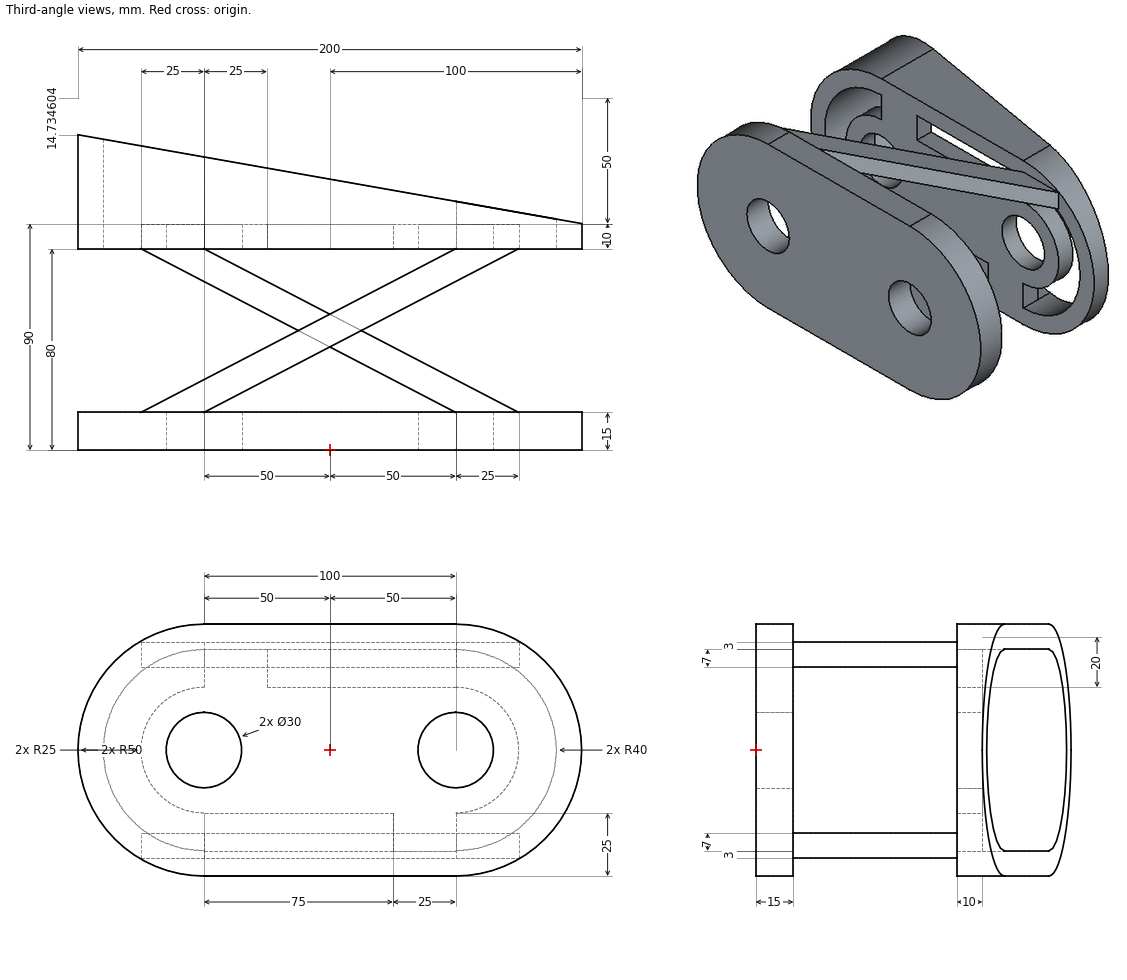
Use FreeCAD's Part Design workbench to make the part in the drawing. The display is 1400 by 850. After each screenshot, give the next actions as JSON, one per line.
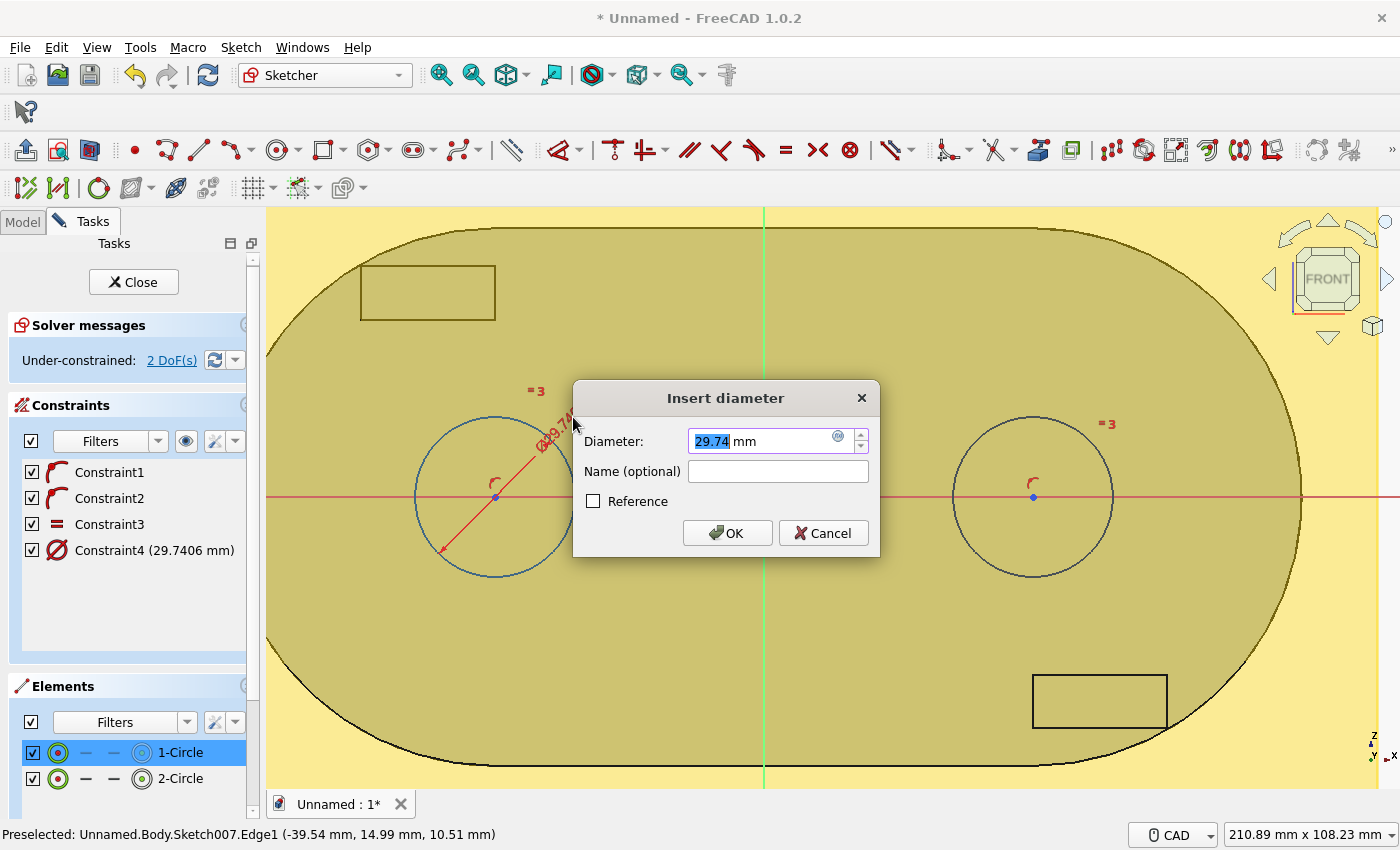
{"action": "type", "text": "30"}
{"action": "key", "text": "Return"}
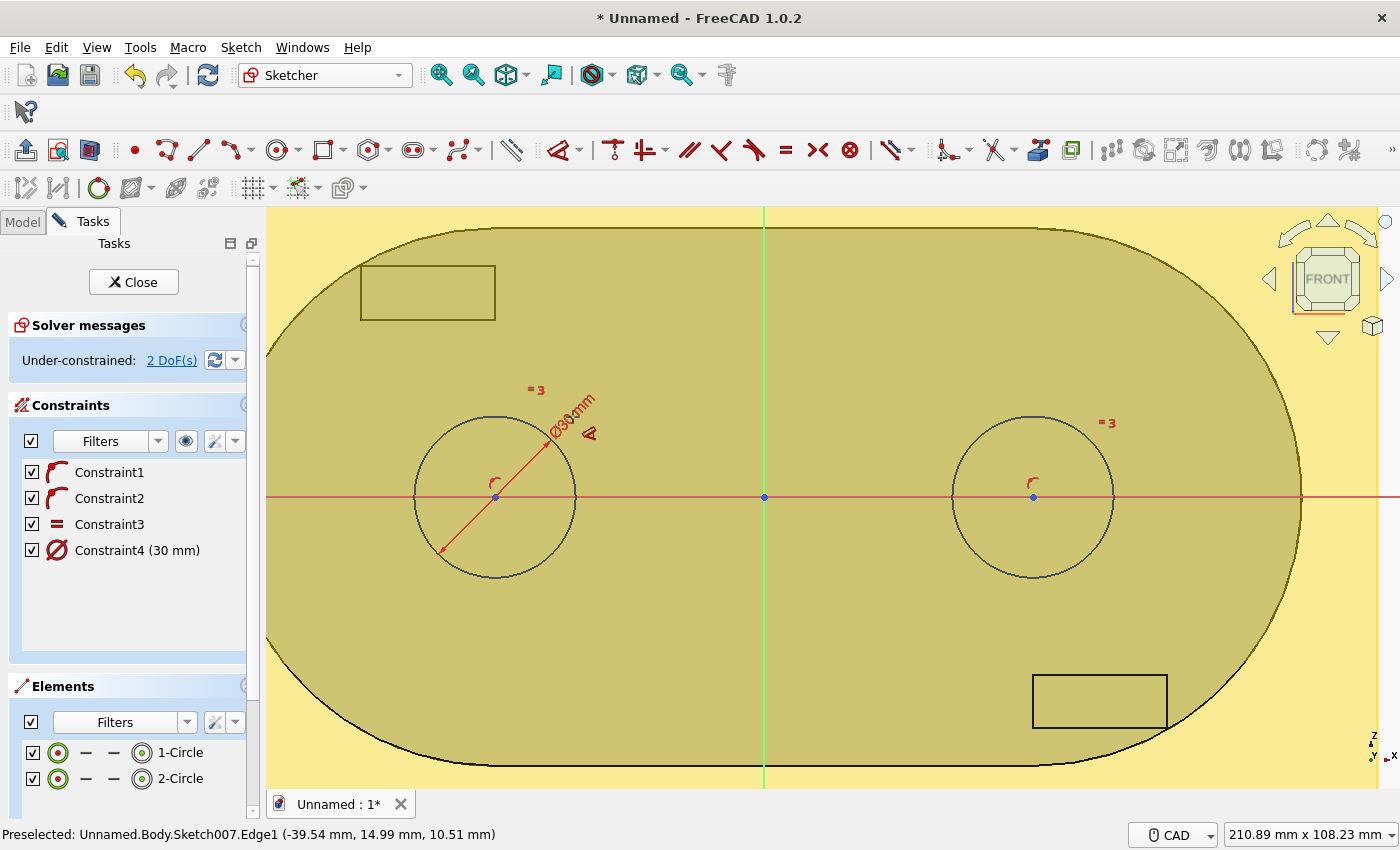
{"action": "left_click", "coordinate": [495, 497]}
{"action": "left_click", "coordinate": [630, 531]}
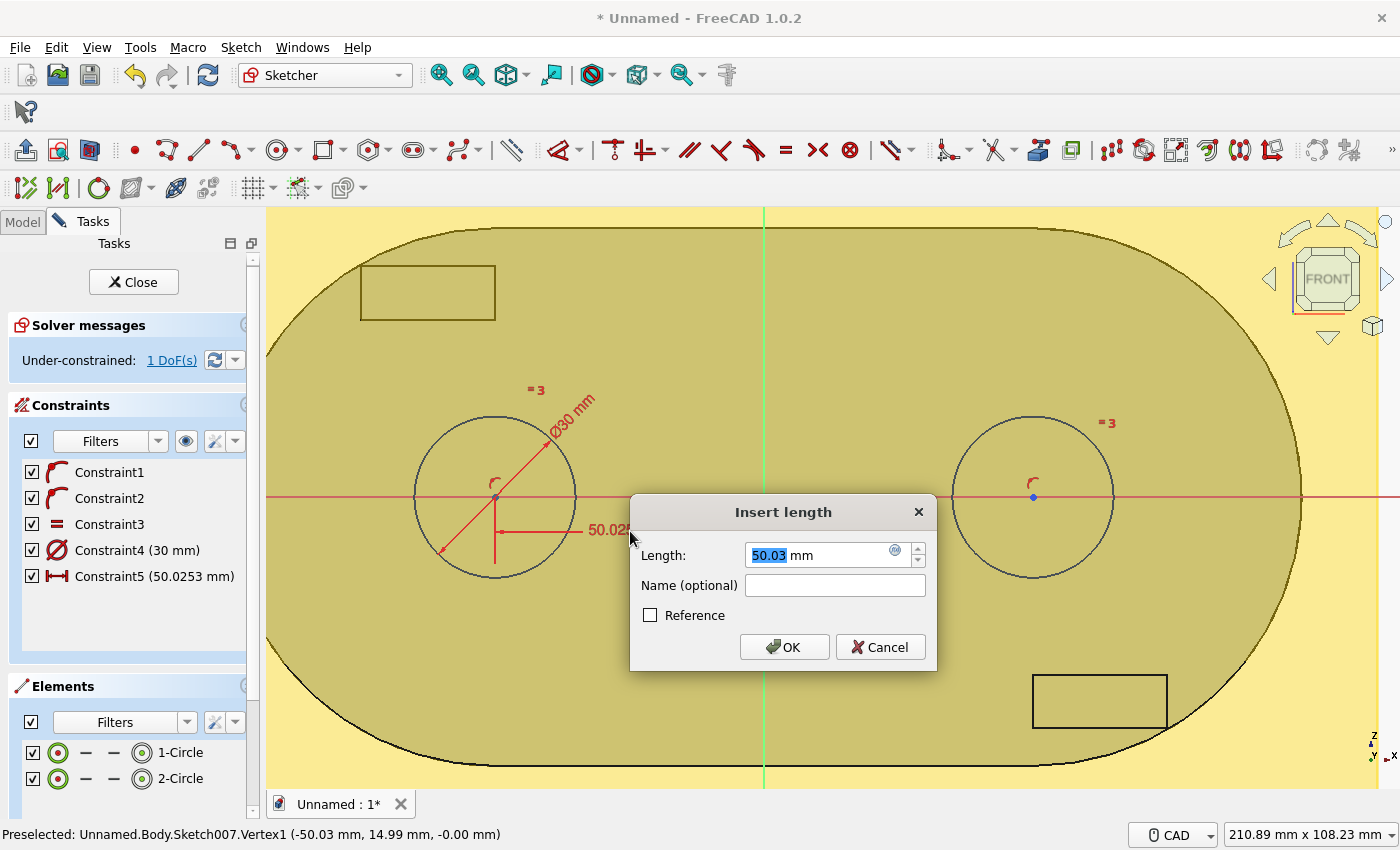
{"action": "type", "text": "50"}
{"action": "key", "text": "Return"}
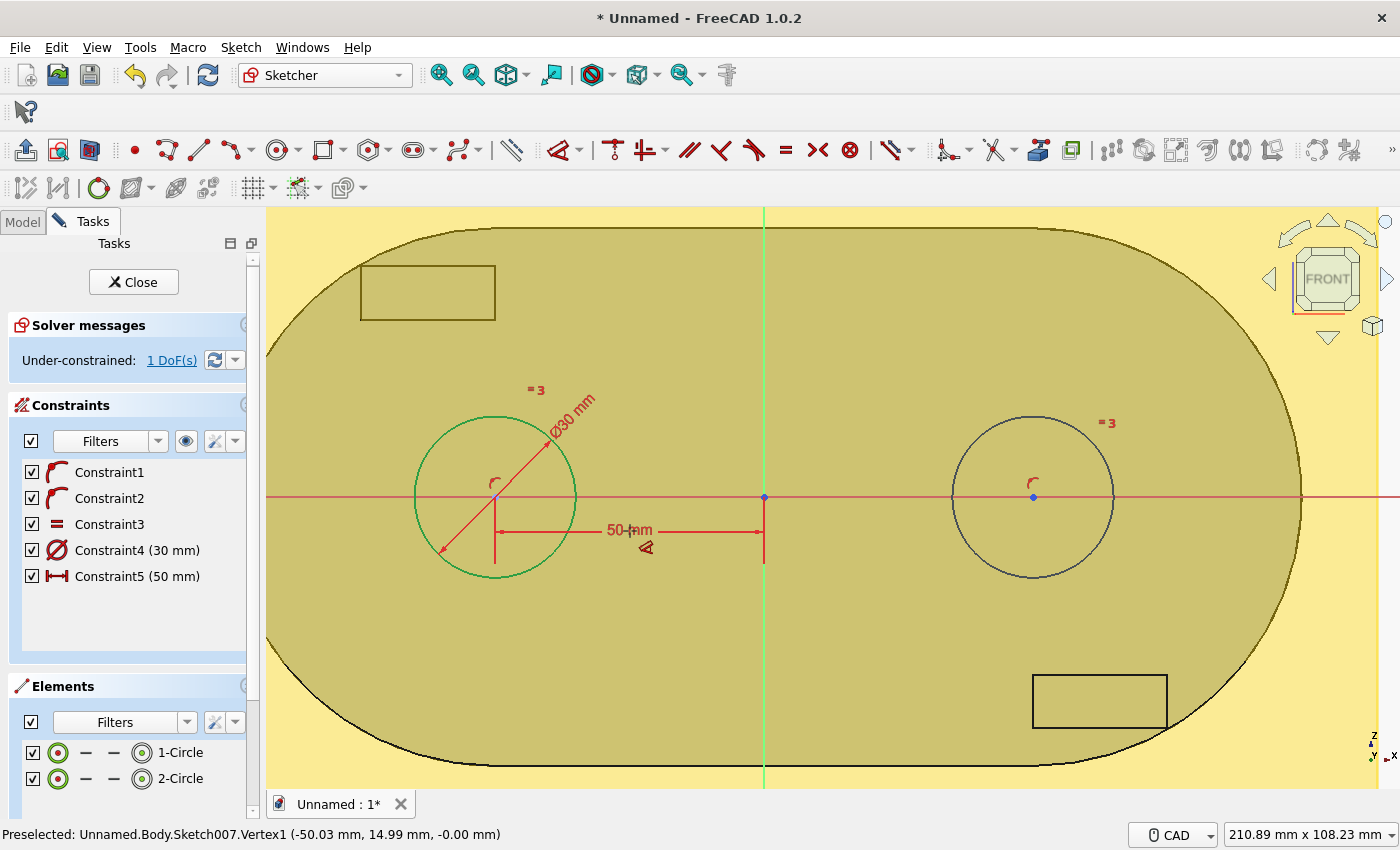
{"action": "left_click", "coordinate": [1033, 497]}
{"action": "left_click", "coordinate": [899, 531]}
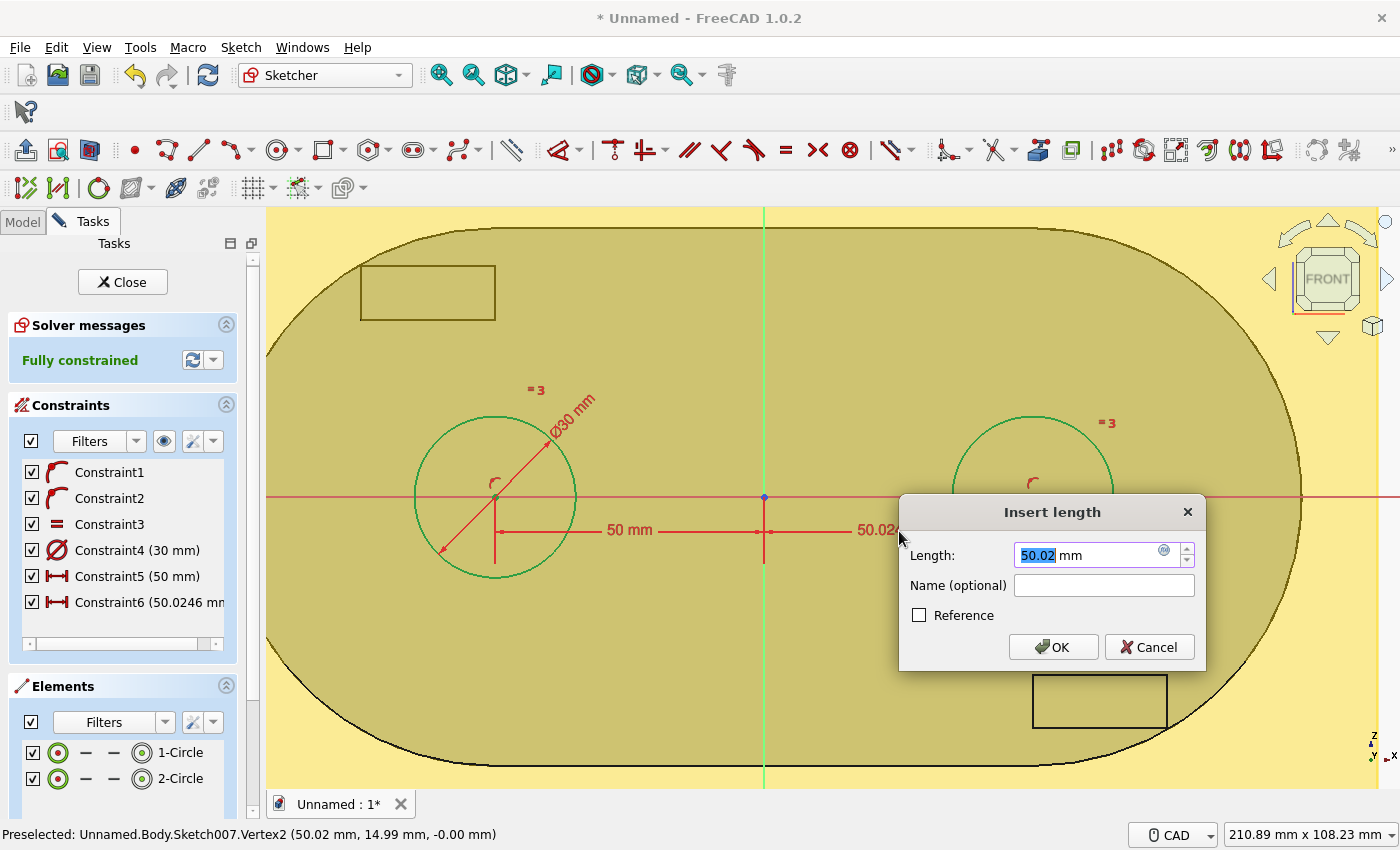
{"action": "type", "text": "50"}
{"action": "key", "text": "Return"}
{"action": "key", "text": "Escape"}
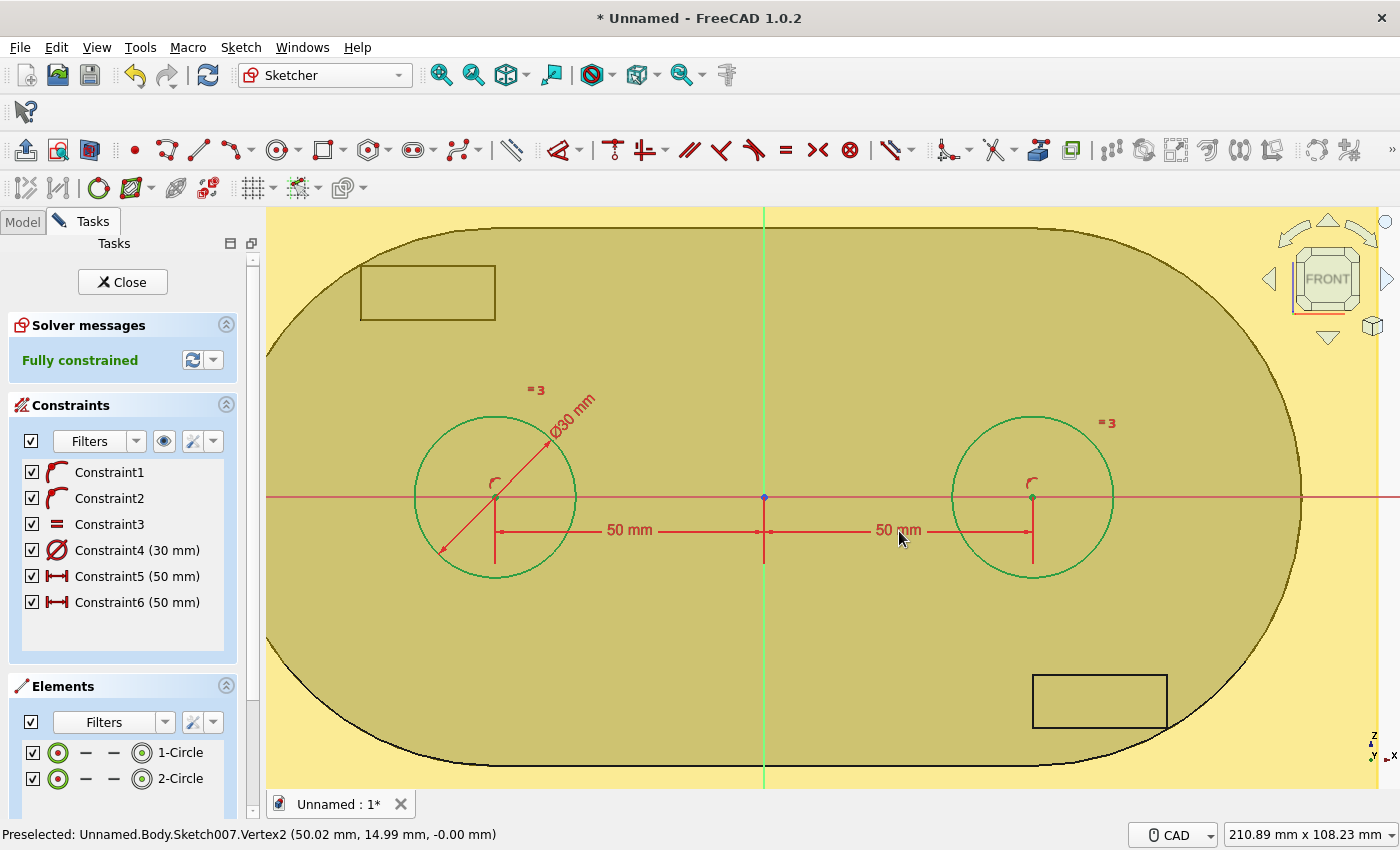
{"action": "left_click", "coordinate": [123, 282]}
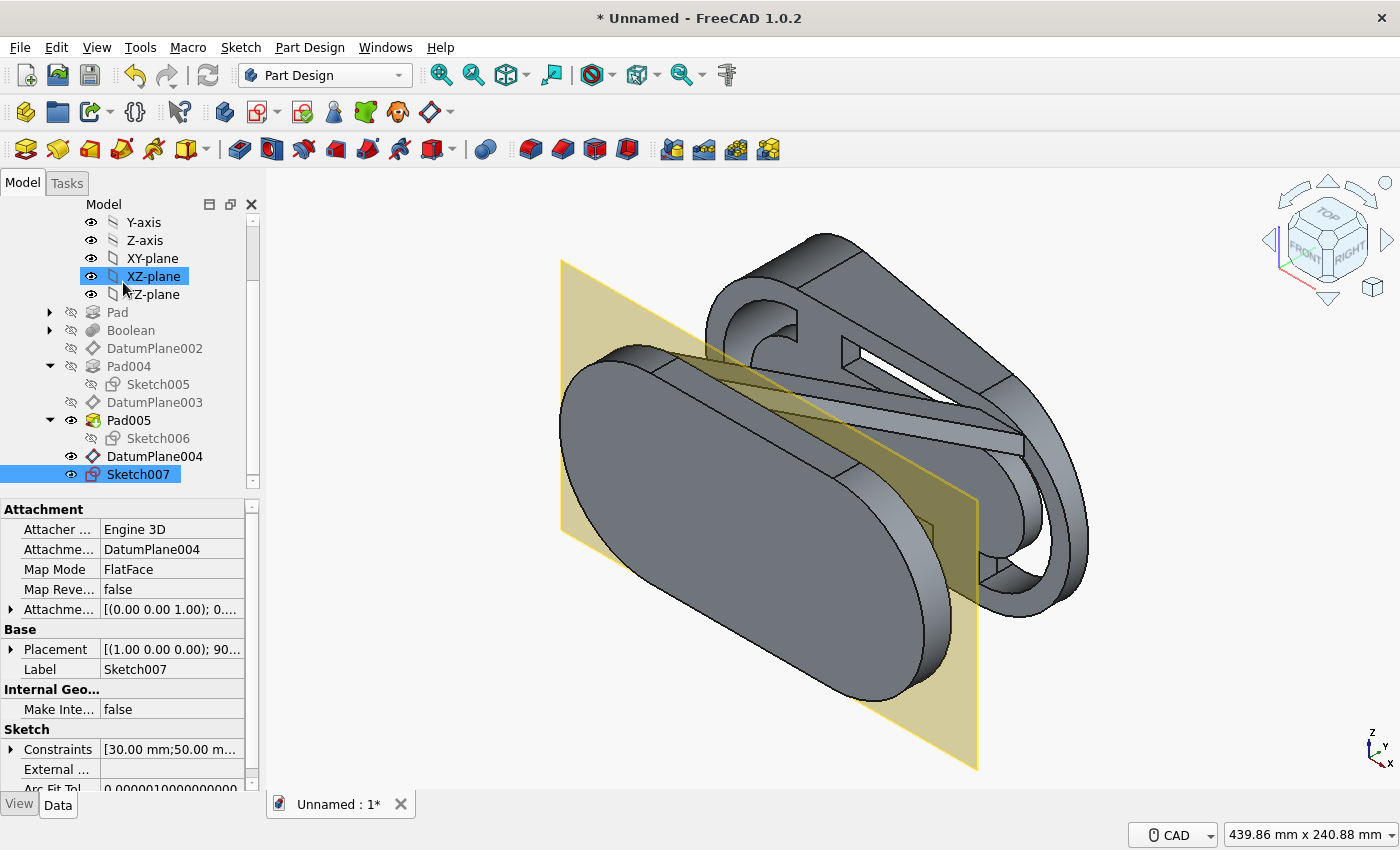
{"action": "left_click", "coordinate": [240, 150]}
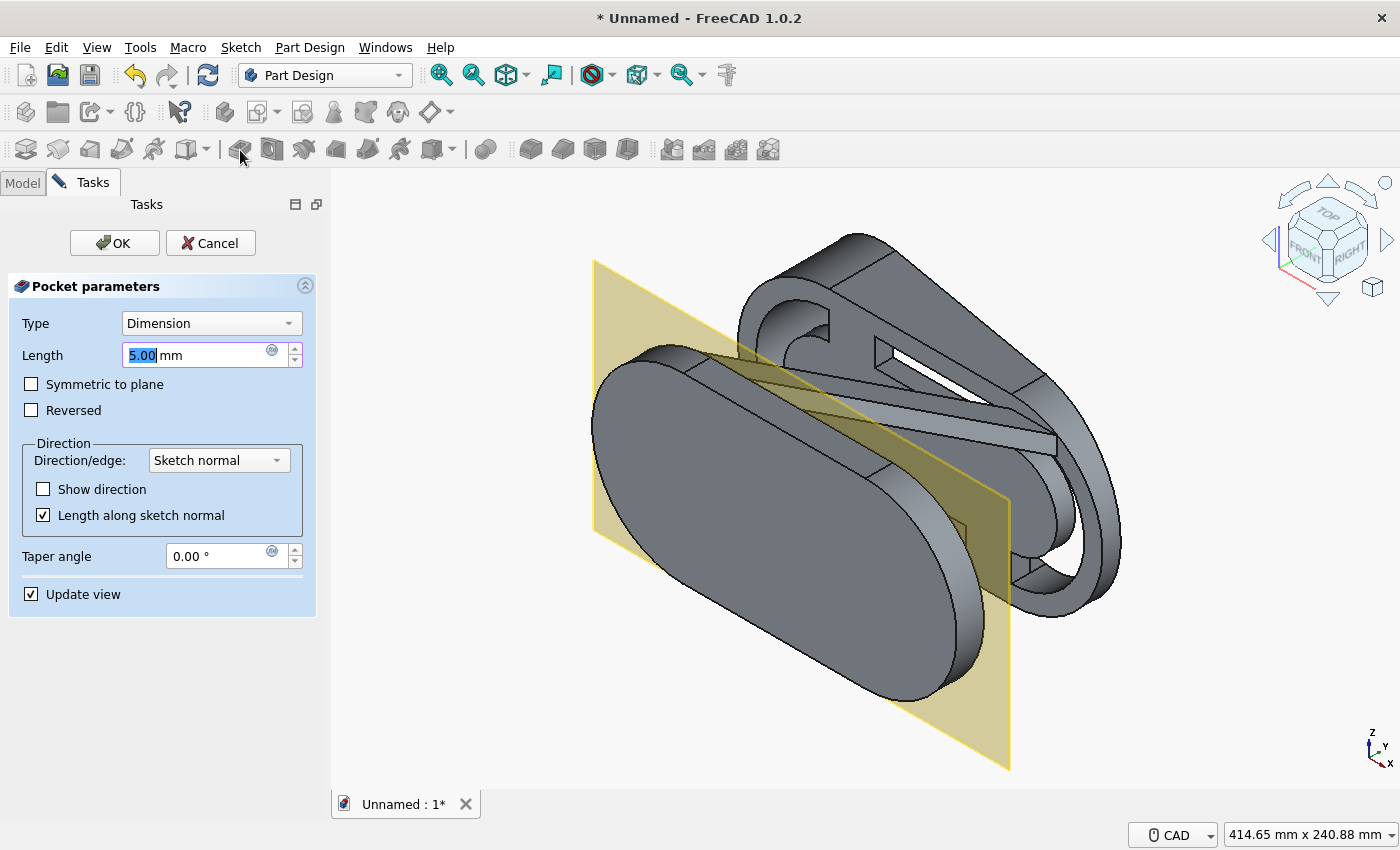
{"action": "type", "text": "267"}
{"action": "key", "text": "Tab"}